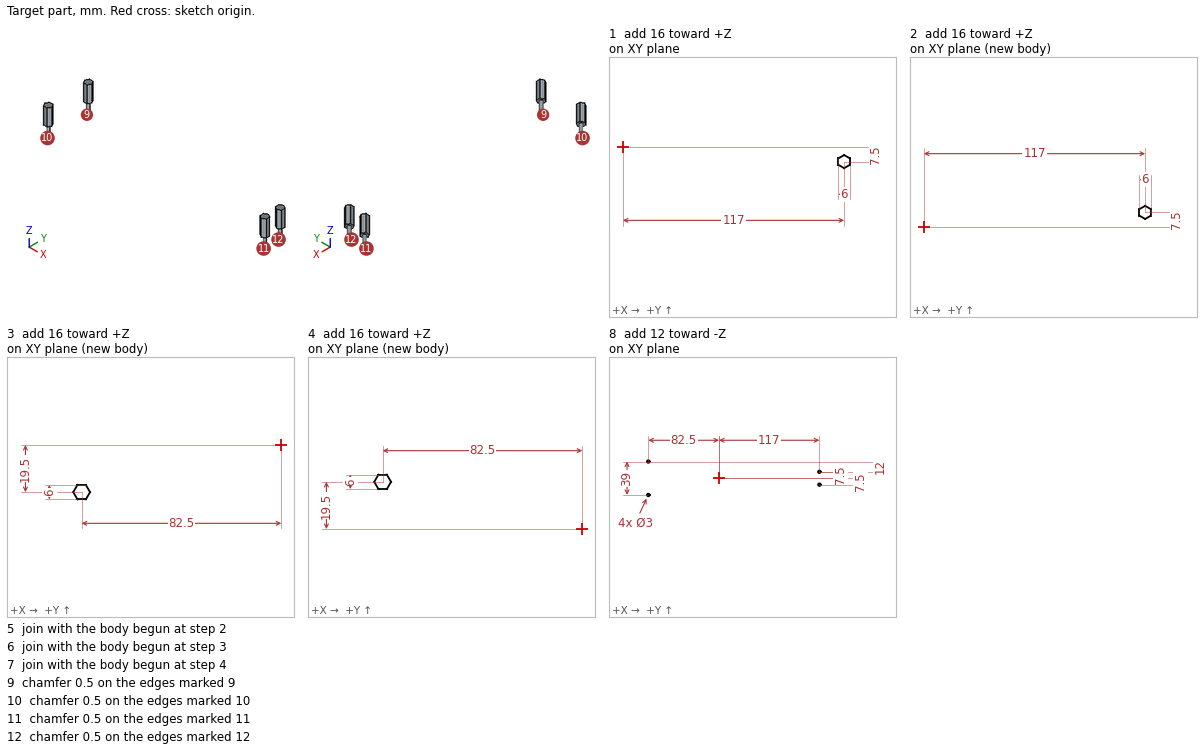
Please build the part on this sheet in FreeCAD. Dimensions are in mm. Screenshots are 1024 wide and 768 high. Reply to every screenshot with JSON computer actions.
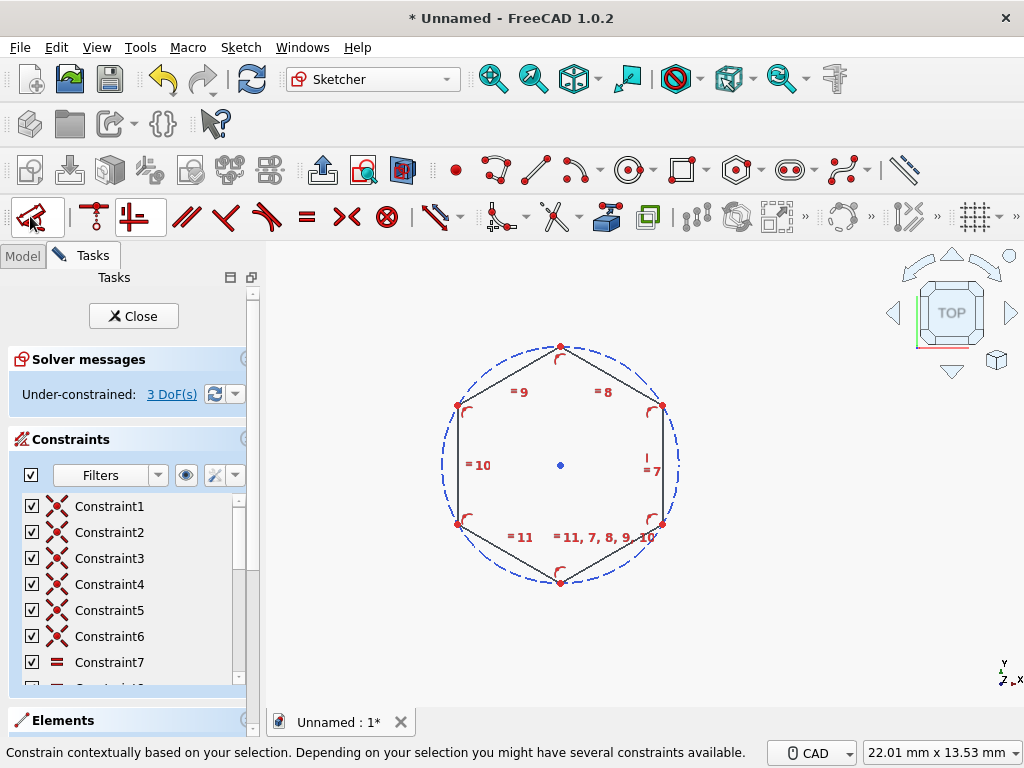
{"action": "left_click", "coordinate": [458, 406]}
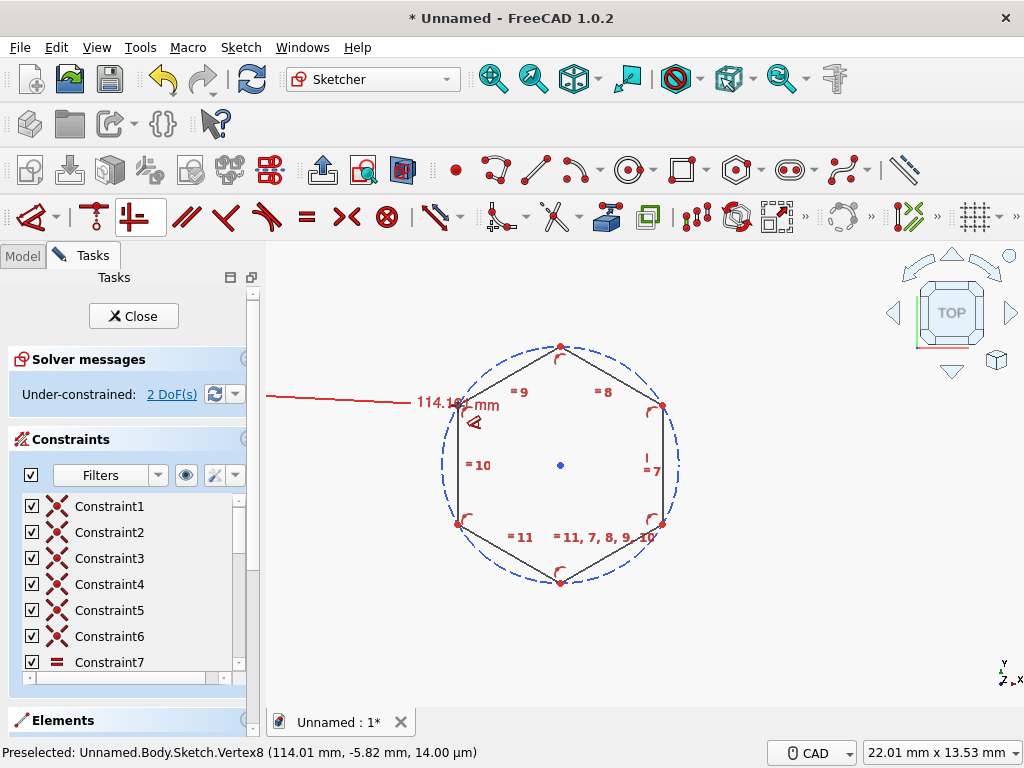
{"action": "left_click", "coordinate": [663, 524]}
{"action": "left_click", "coordinate": [560, 558]}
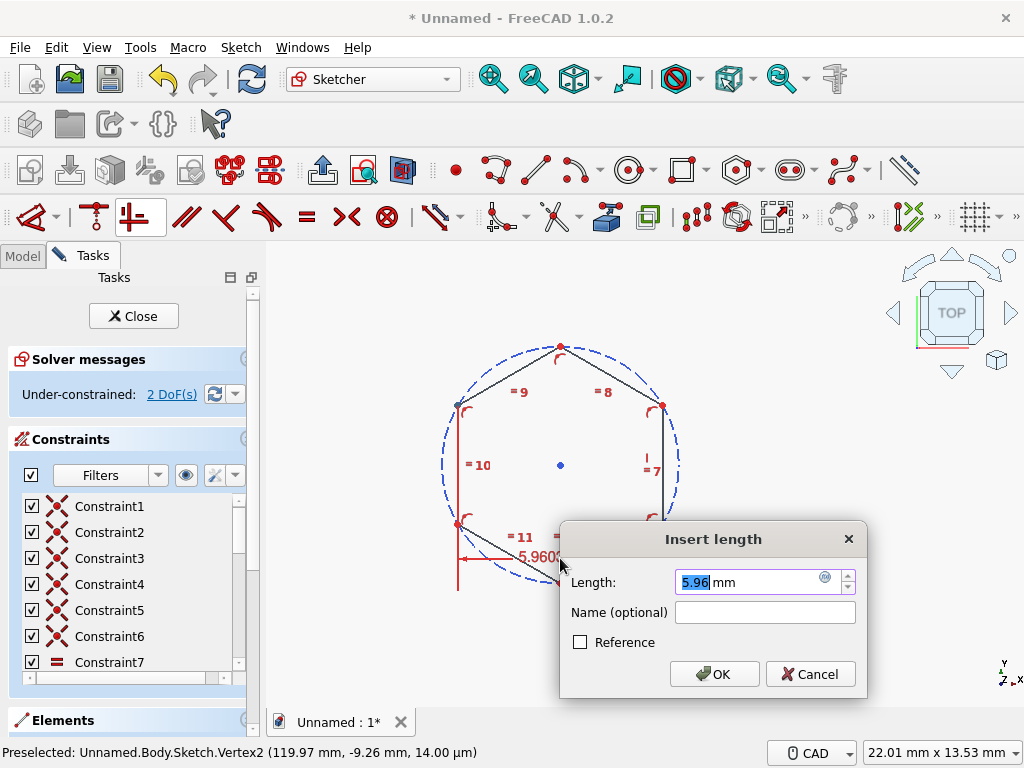
{"action": "type", "text": "6"}
{"action": "key", "text": "Return"}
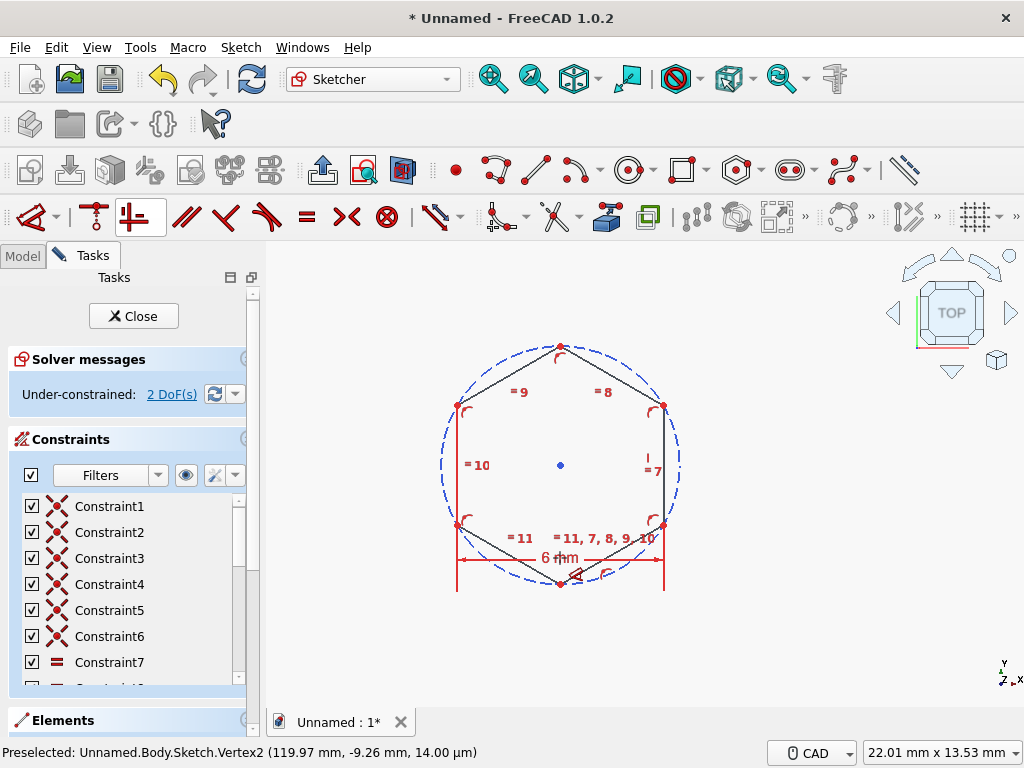
{"action": "left_click", "coordinate": [560, 465]}
{"action": "left_click", "coordinate": [427, 499]}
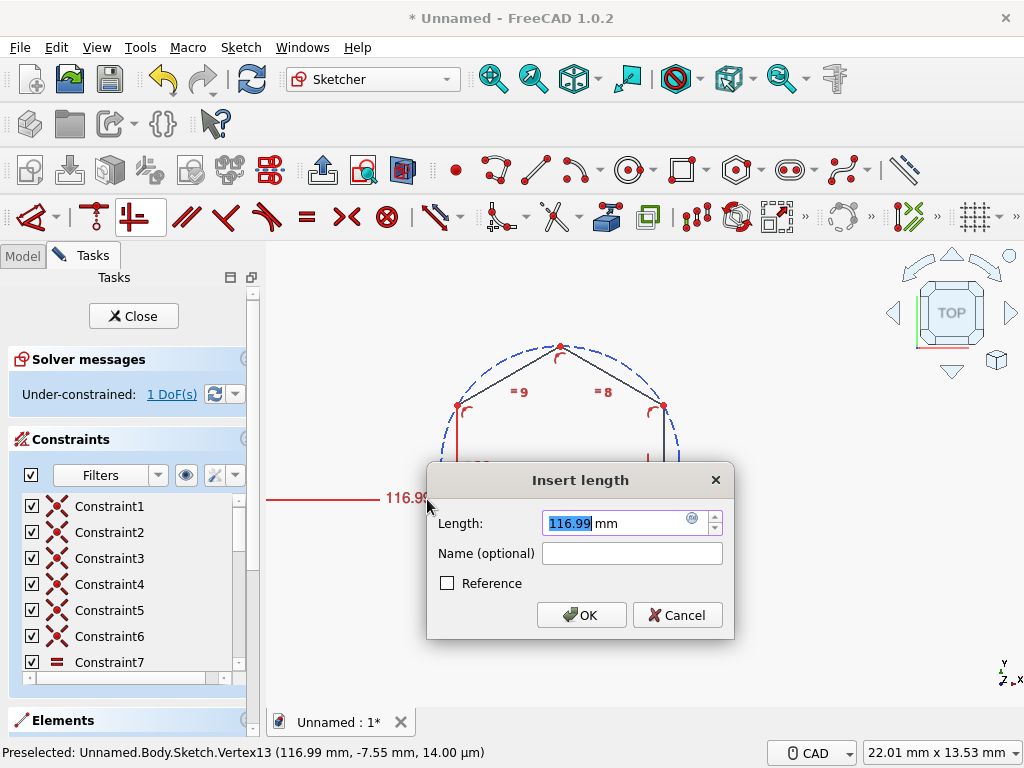
{"action": "type", "text": "117"}
{"action": "key", "text": "Return"}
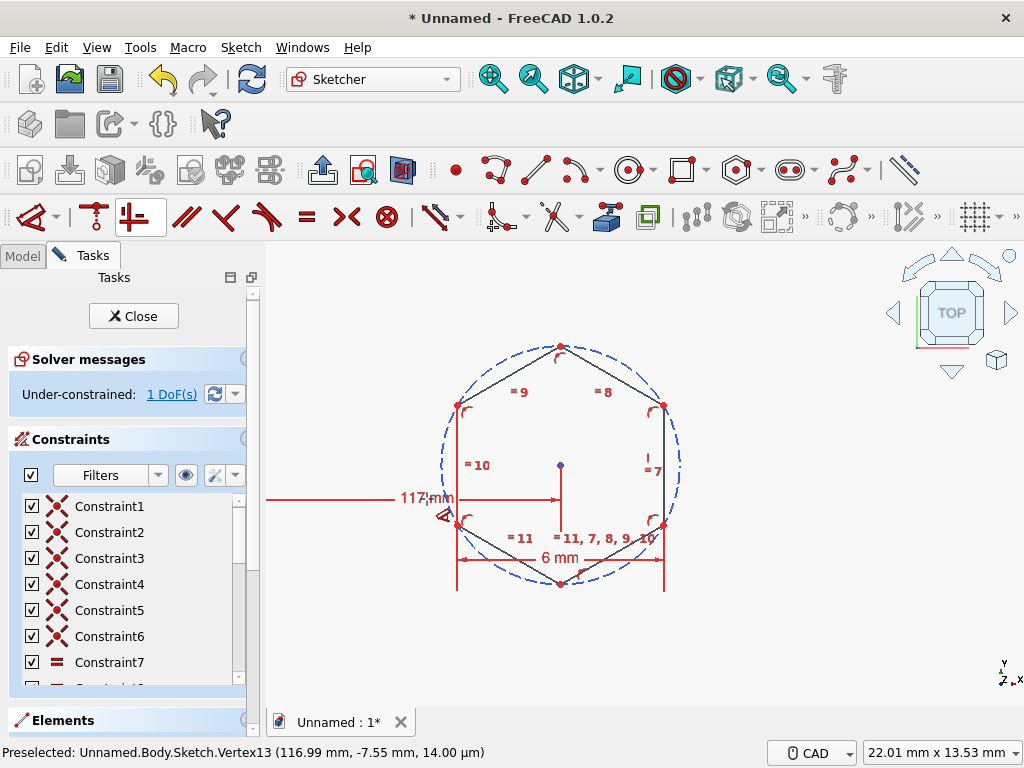
{"action": "left_click", "coordinate": [561, 465]}
{"action": "left_click", "coordinate": [595, 322]}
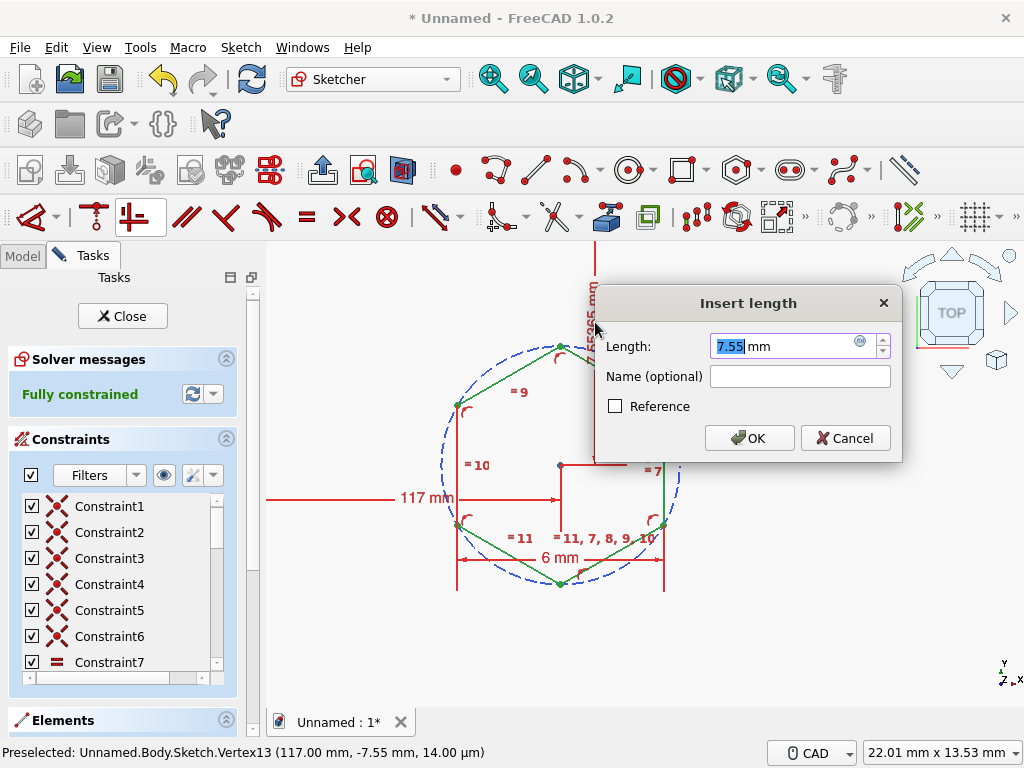
{"action": "type", "text": "7.5"}
{"action": "key", "text": "Return"}
{"action": "key", "text": "Escape"}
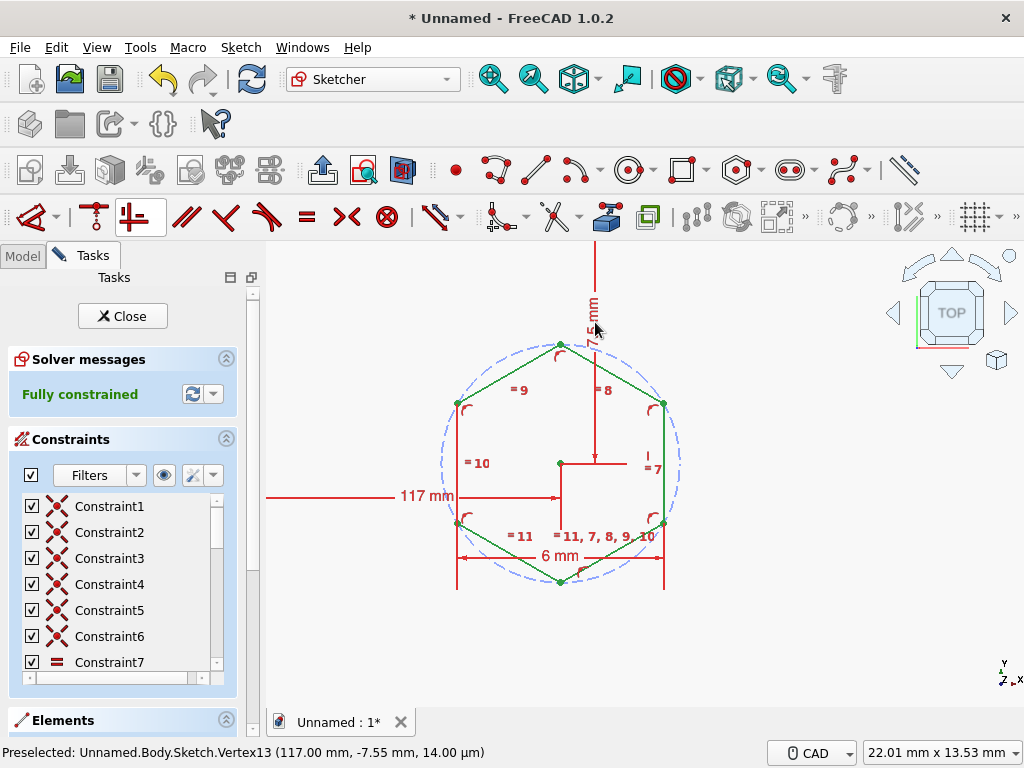
{"action": "left_click", "coordinate": [123, 316]}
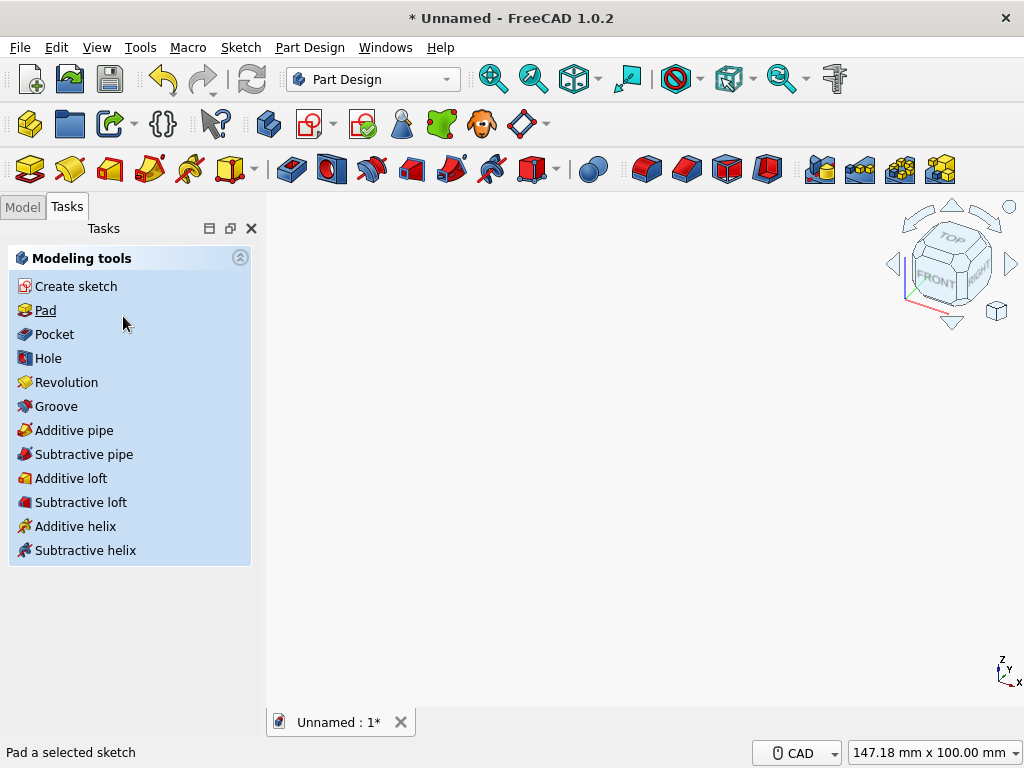
{"action": "left_click", "coordinate": [30, 170]}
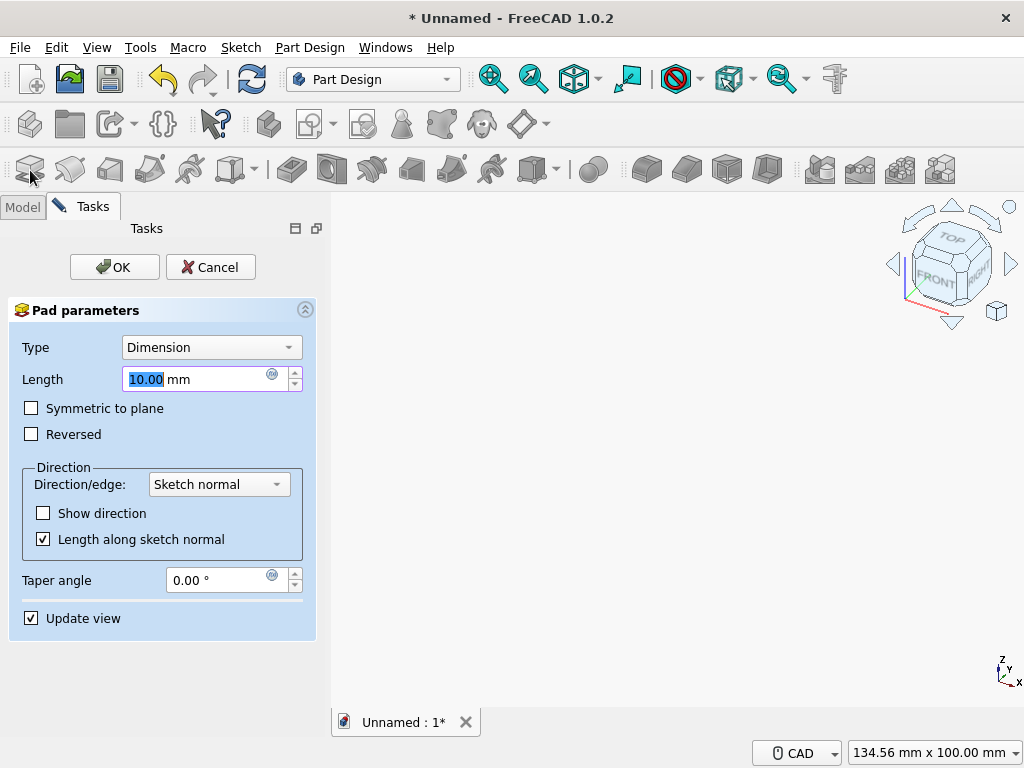
{"action": "type", "text": "16"}
{"action": "key", "text": "Tab"}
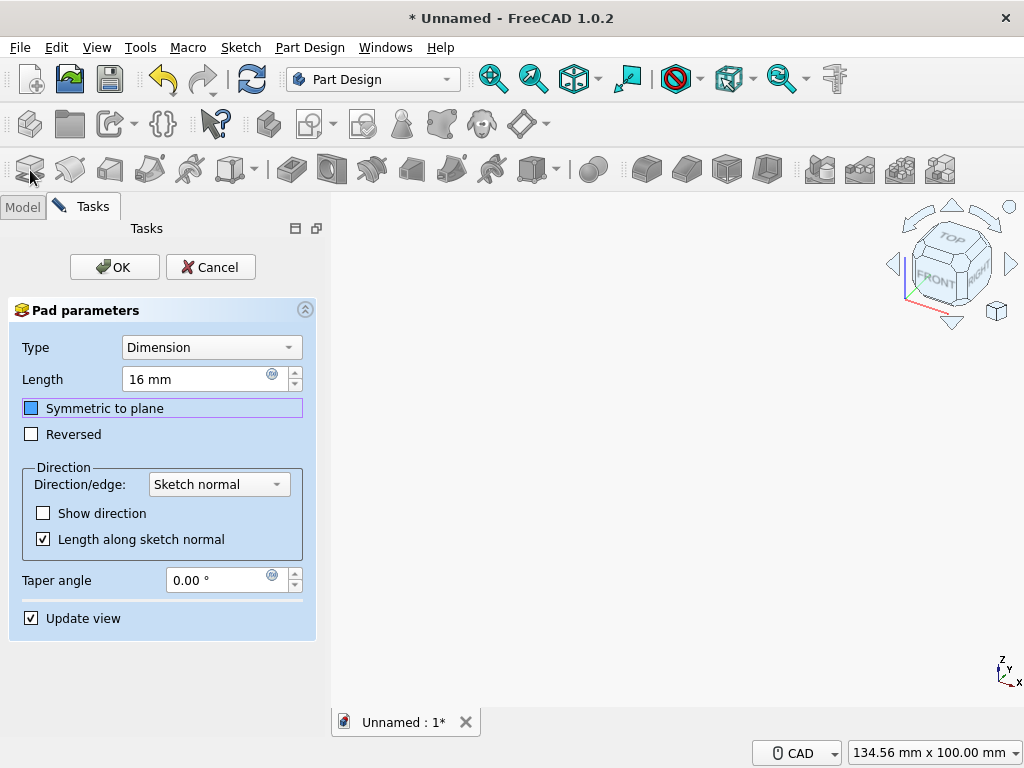
{"action": "left_click", "coordinate": [115, 267]}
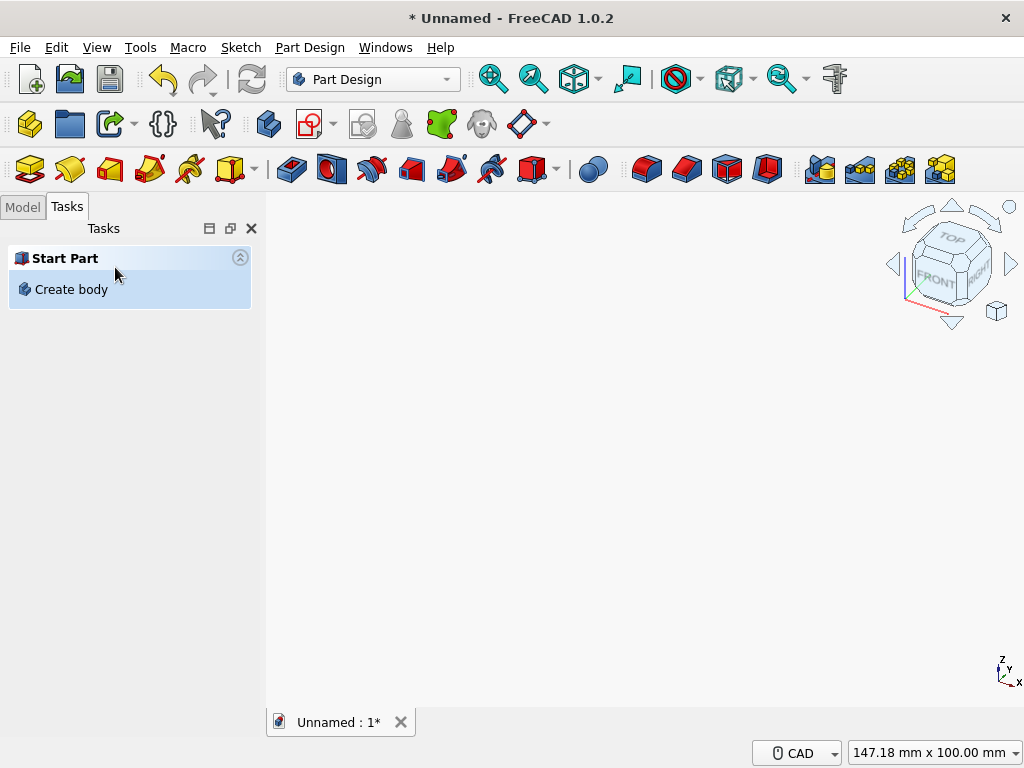
{"action": "left_click", "coordinate": [494, 80]}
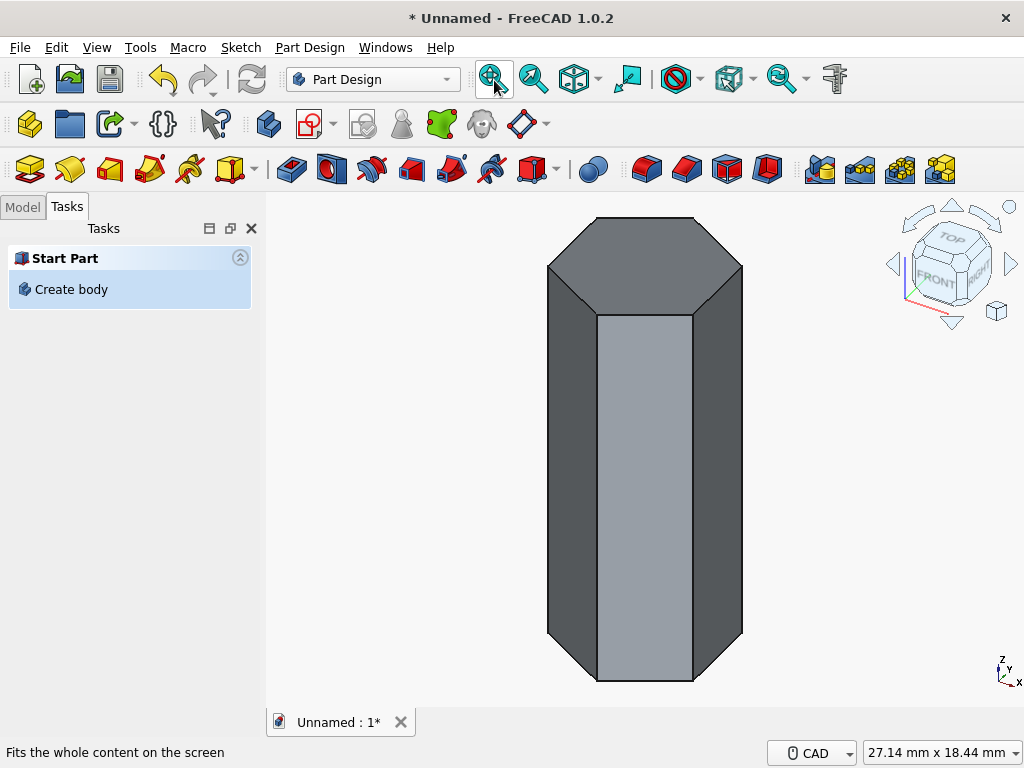
{"action": "left_click", "coordinate": [270, 124]}